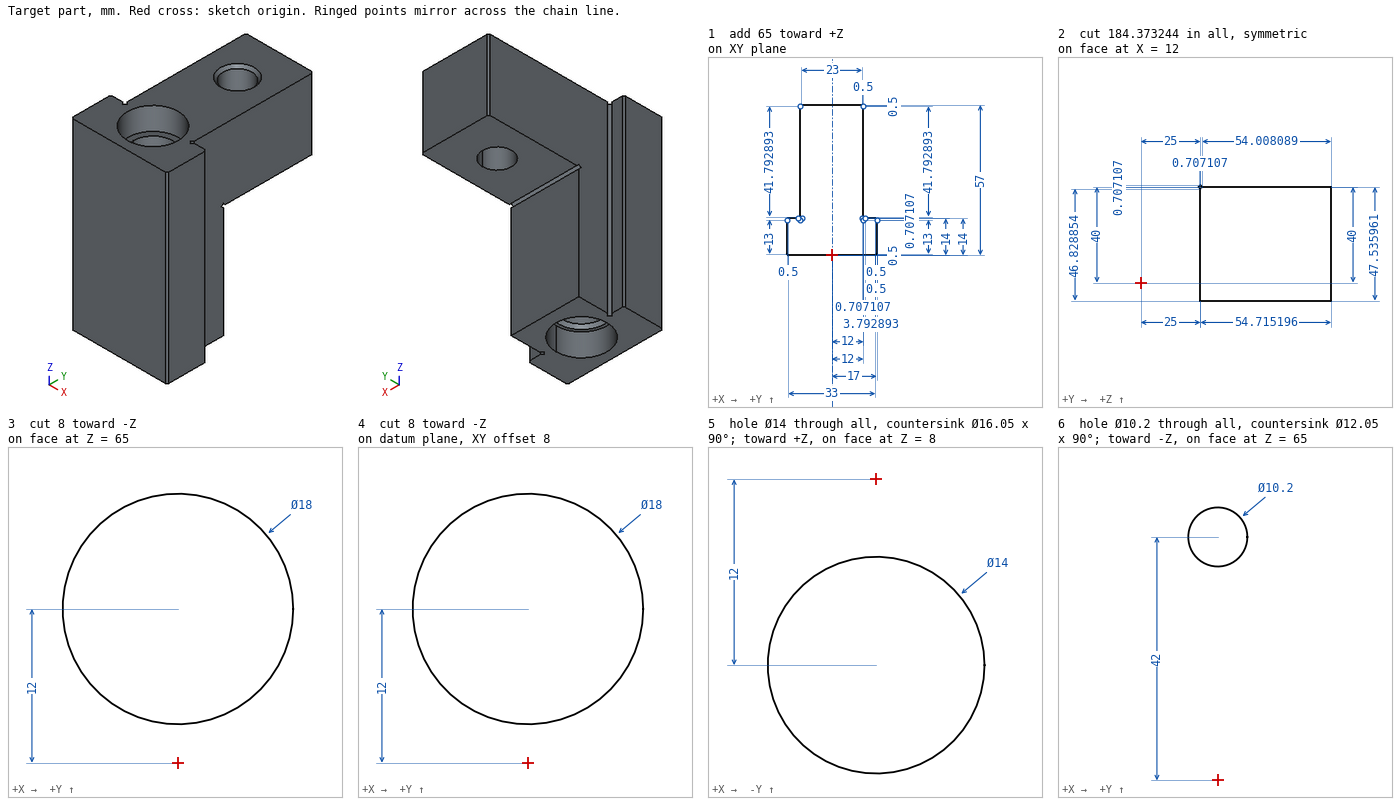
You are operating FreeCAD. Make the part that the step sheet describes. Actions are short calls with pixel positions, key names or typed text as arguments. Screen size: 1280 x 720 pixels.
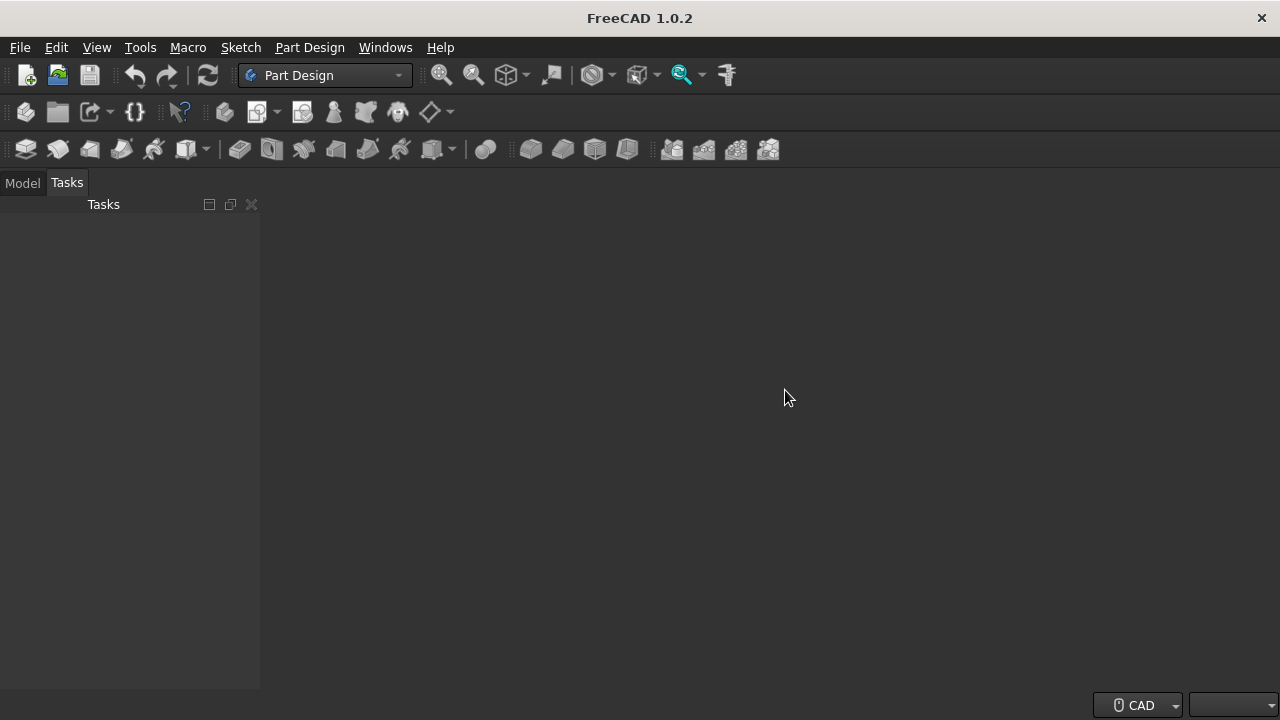
click(26, 76)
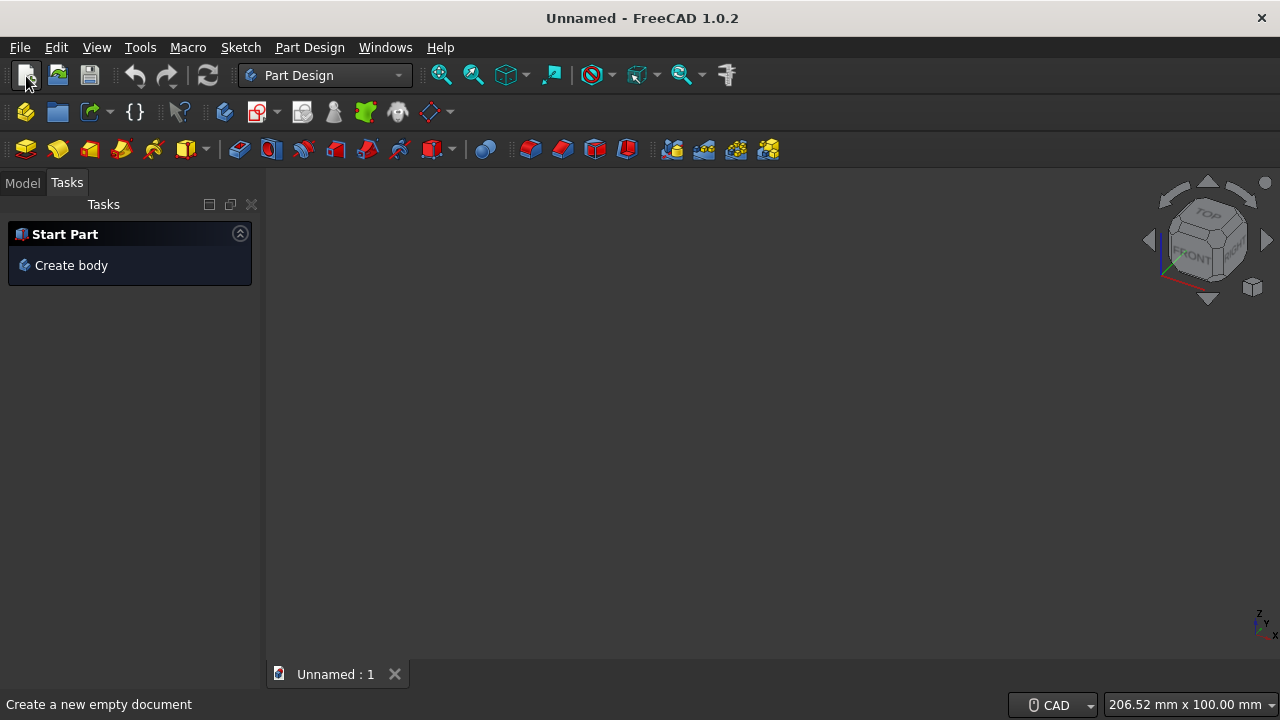
click(258, 112)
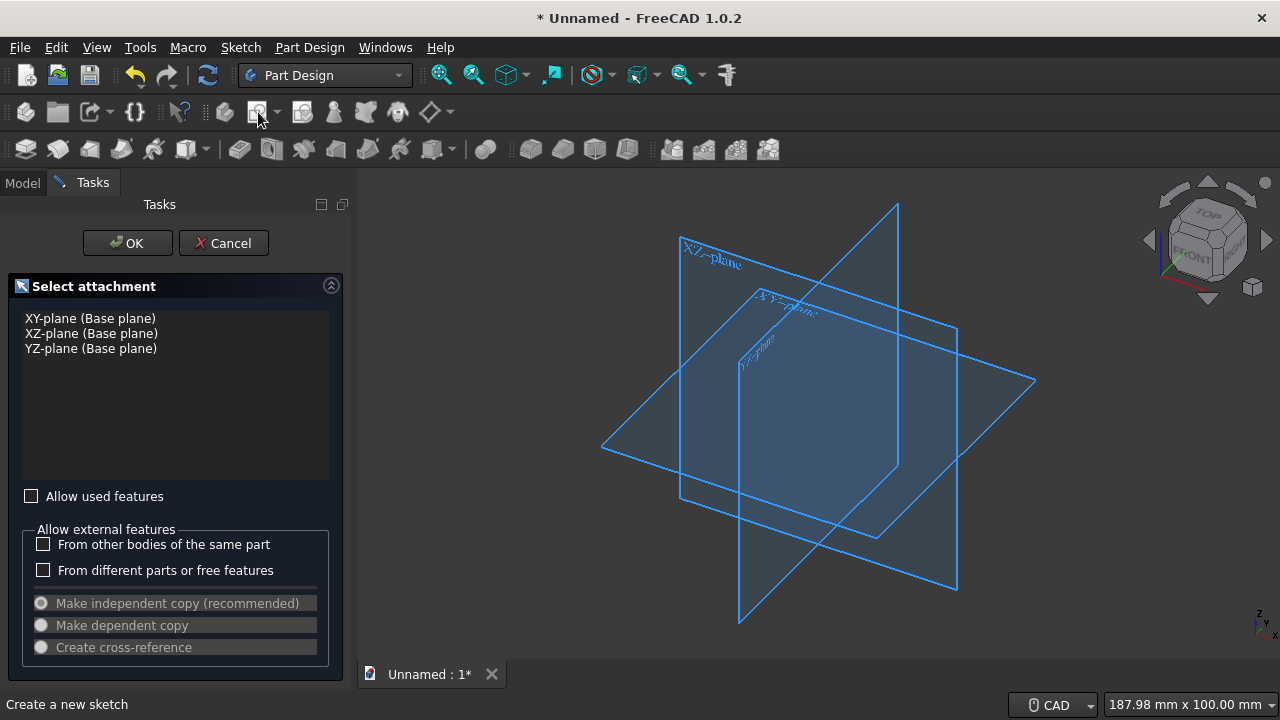
click(82, 318)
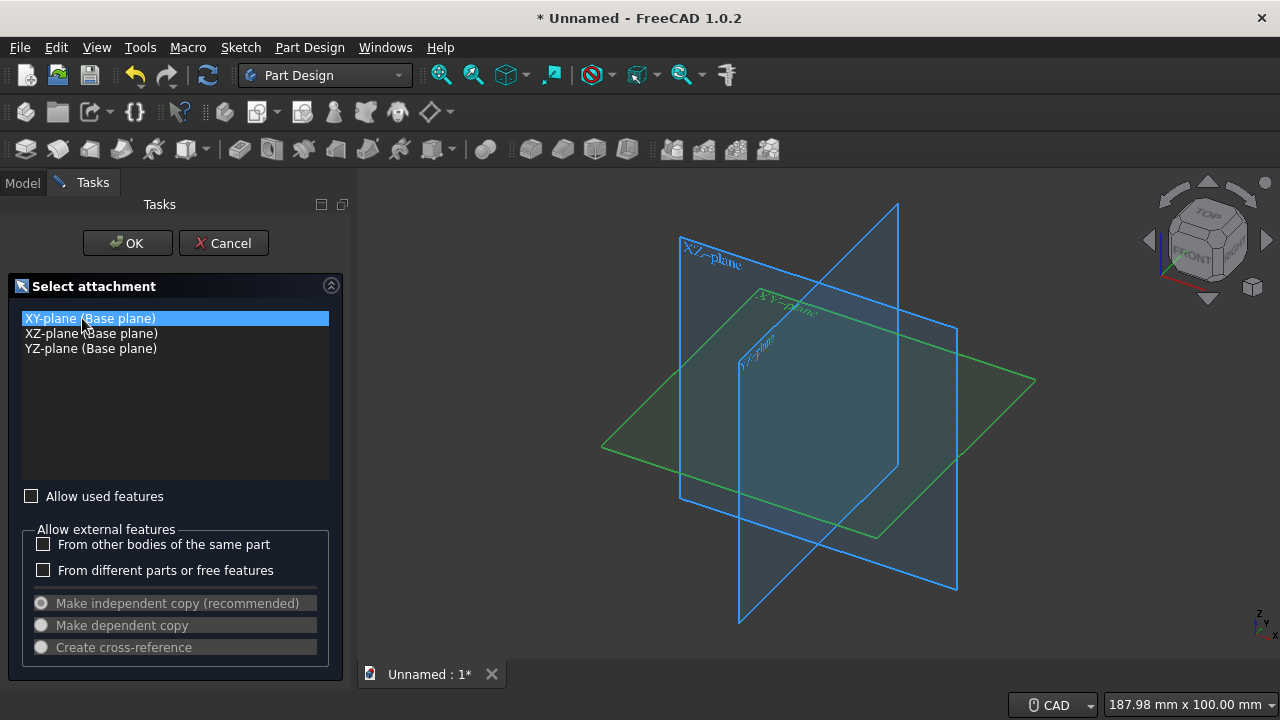
click(128, 243)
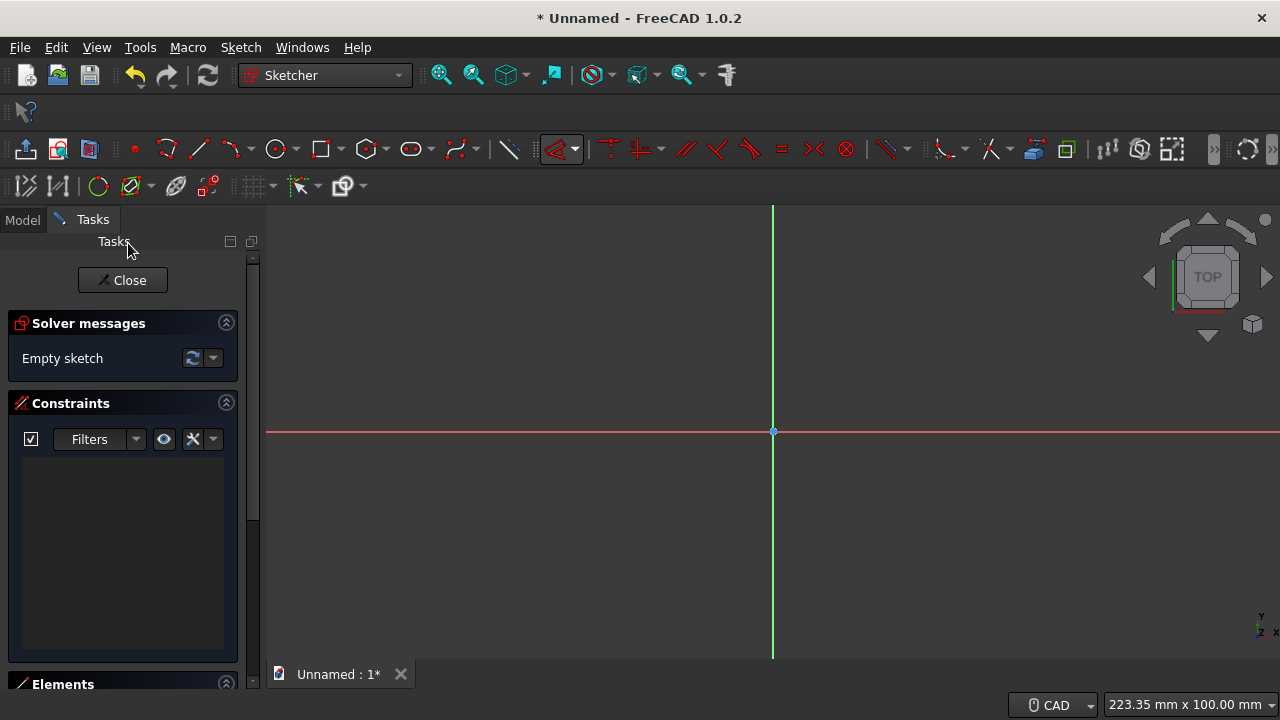
scroll(565, 631, down, 2)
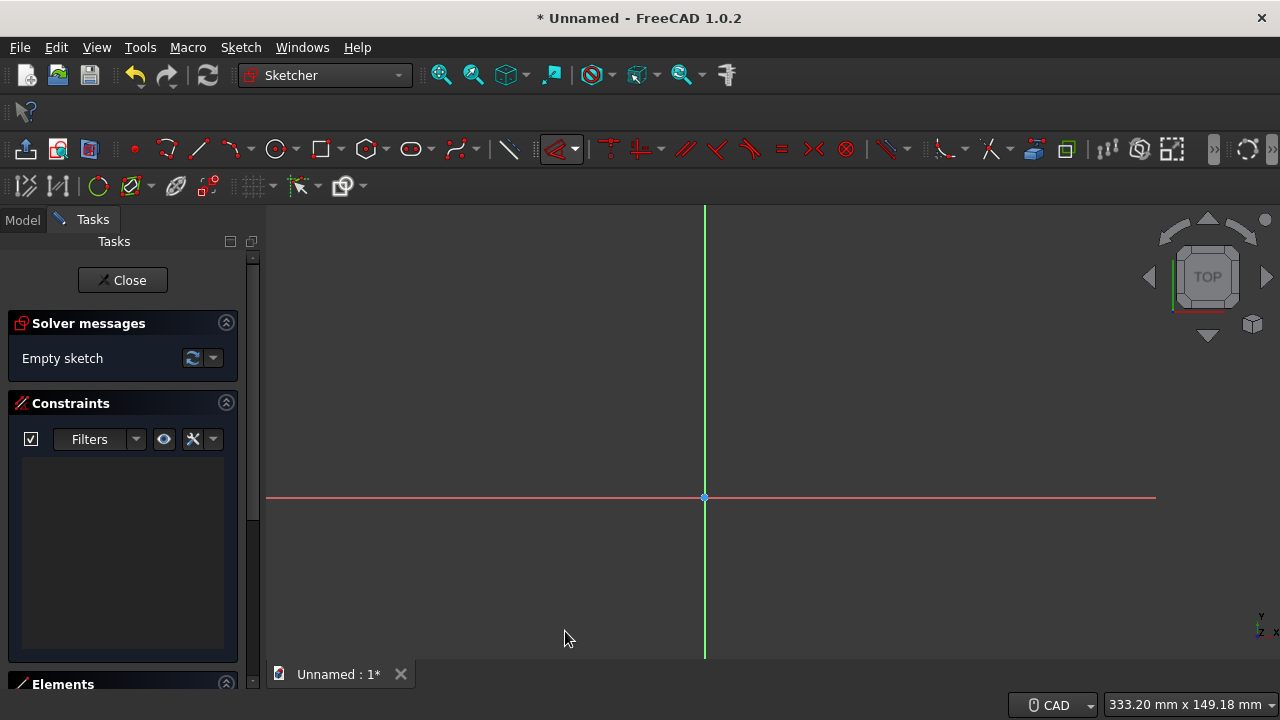
scroll(705, 369, up, 2)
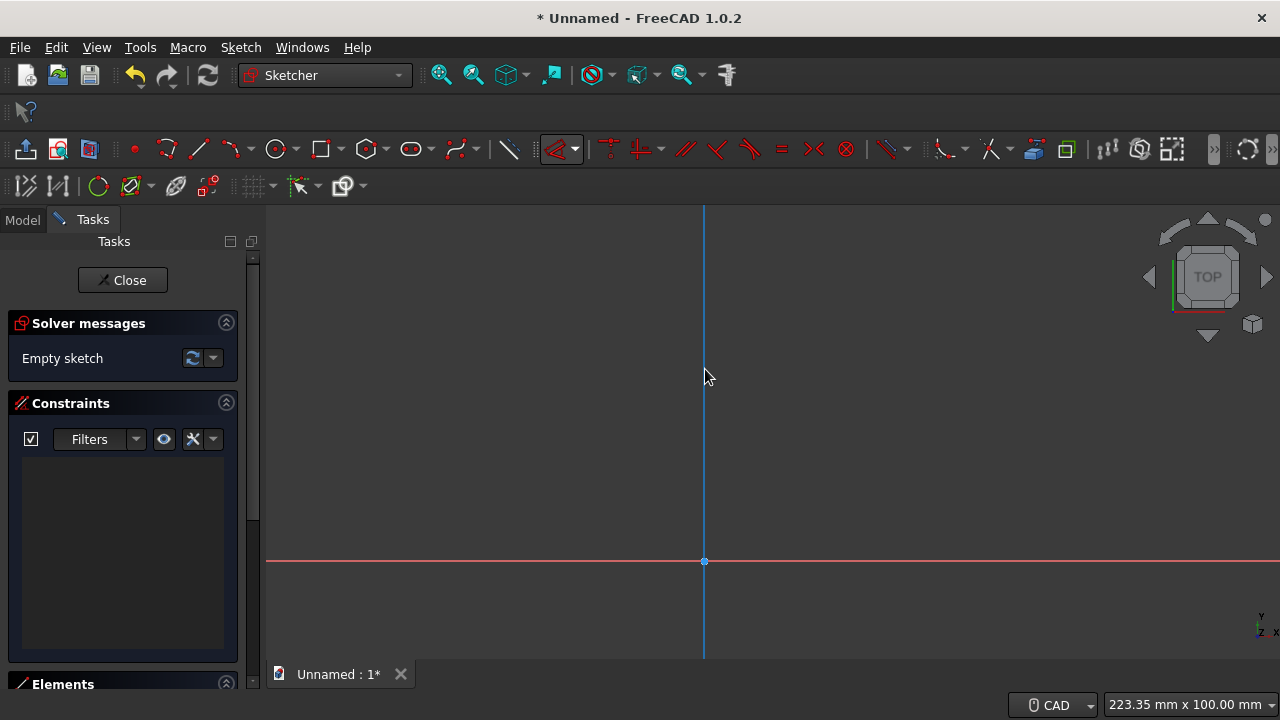
click(168, 150)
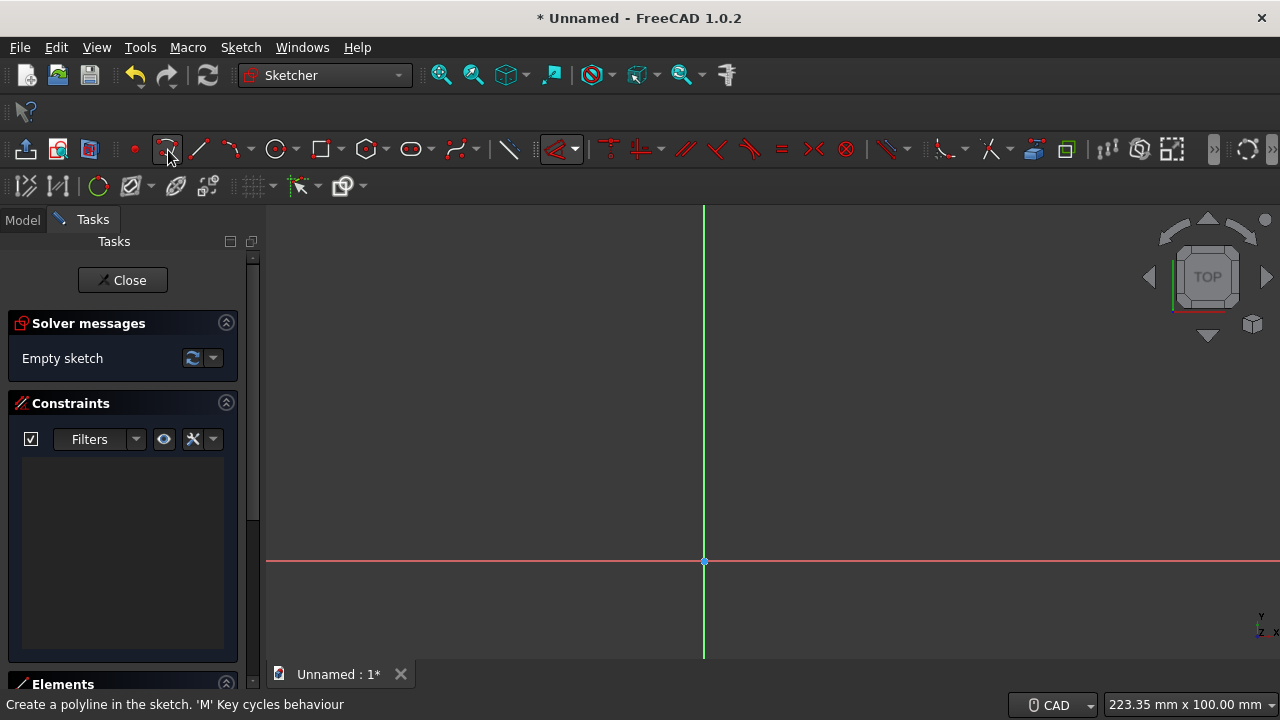
click(629, 561)
click(779, 552)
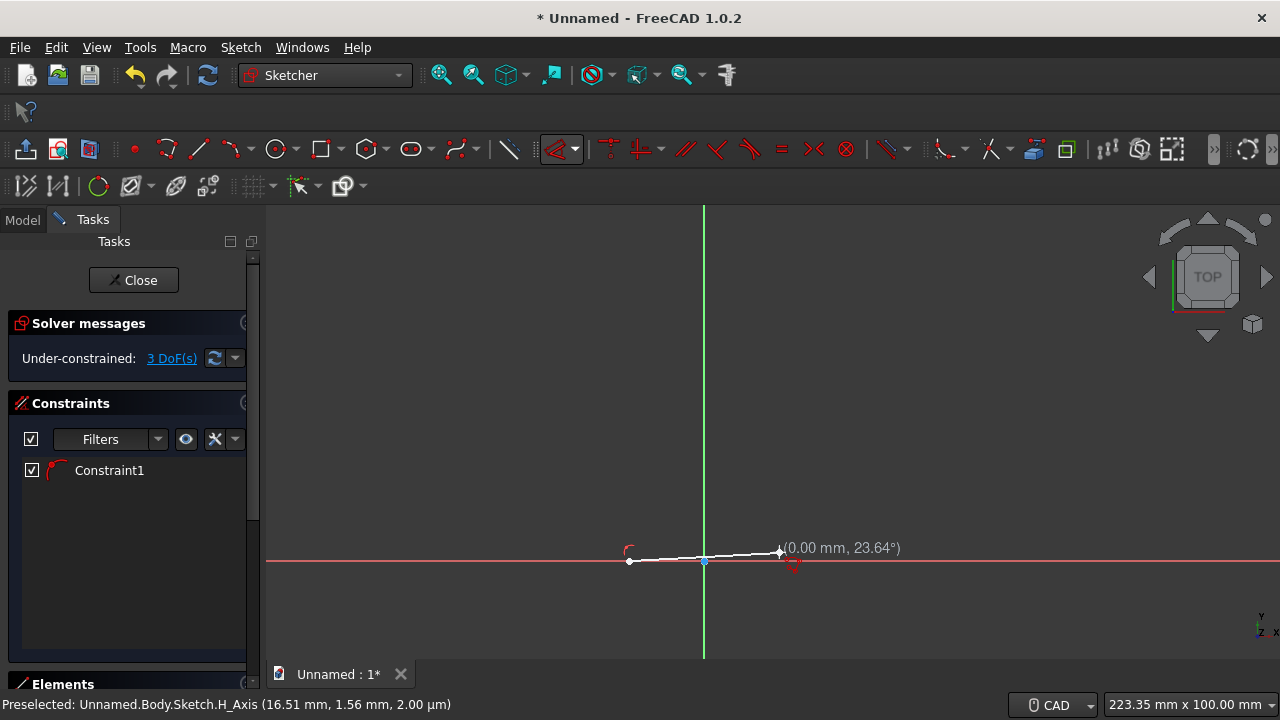
scroll(781, 559, up, 10)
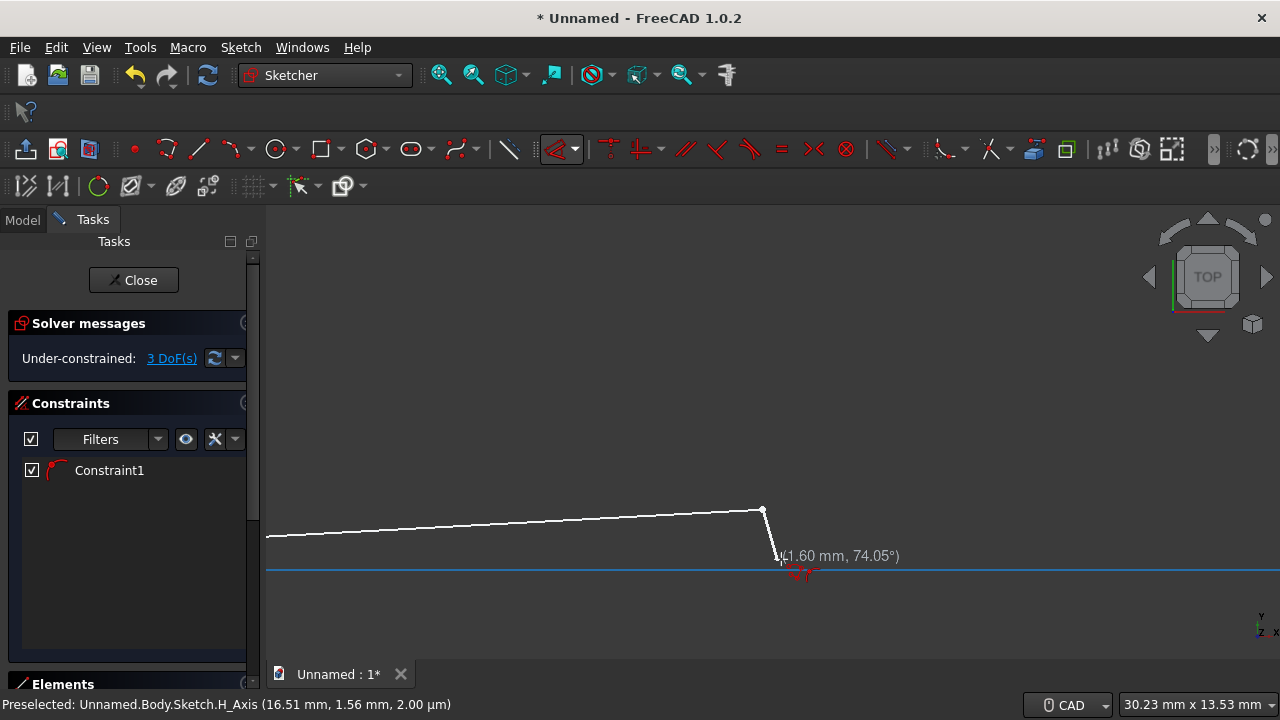
click(780, 553)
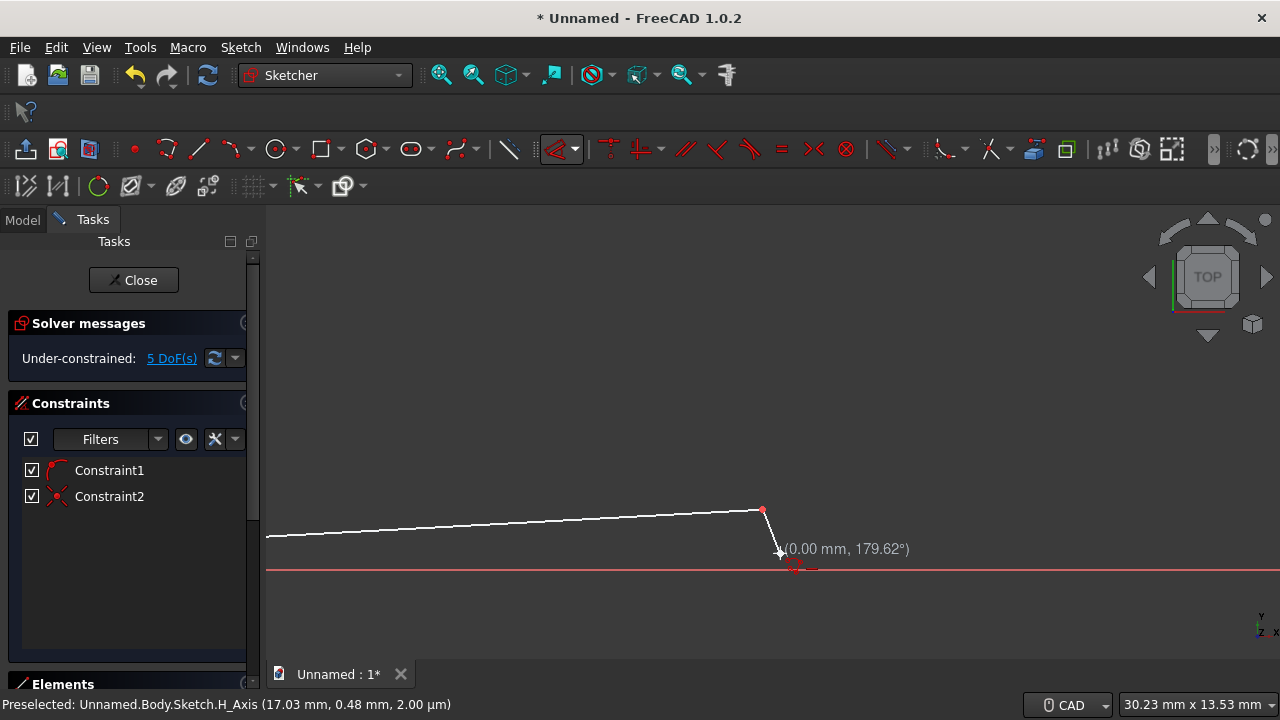
scroll(782, 560, down, 10)